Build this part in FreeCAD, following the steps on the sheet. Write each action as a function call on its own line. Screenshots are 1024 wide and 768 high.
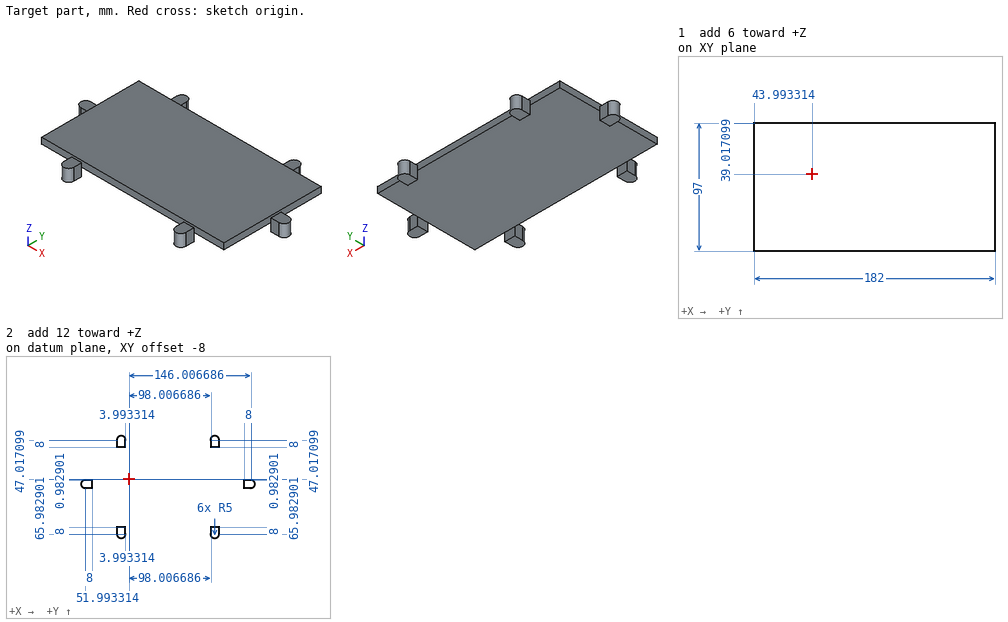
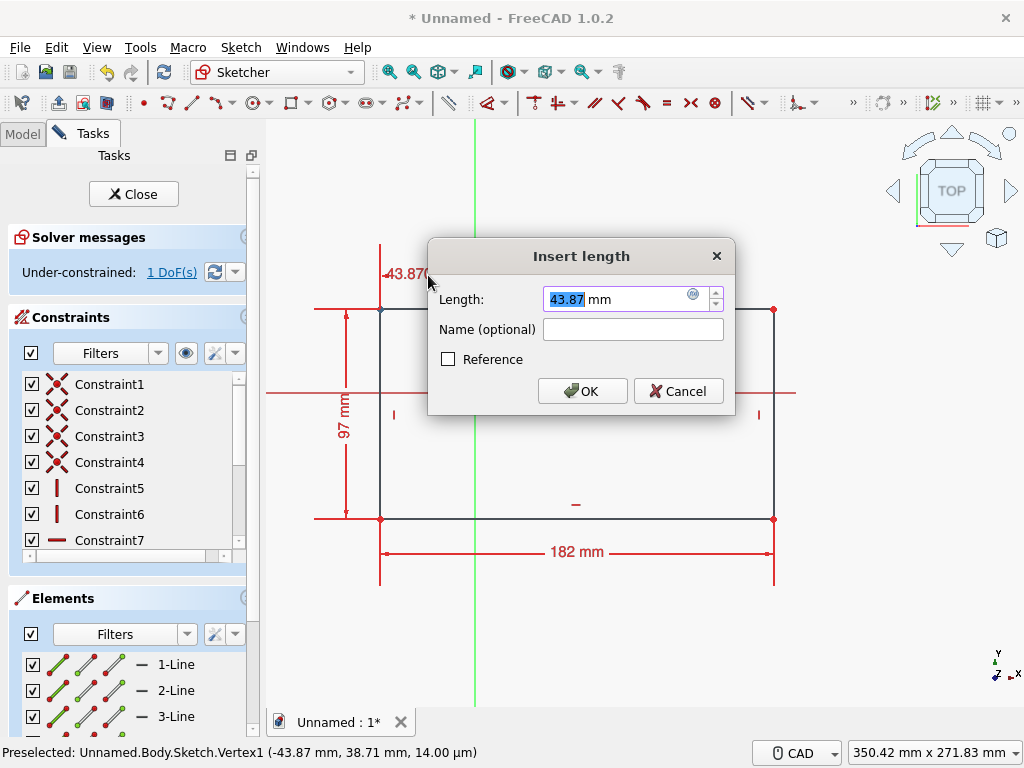
text(43.993314)
key(Return)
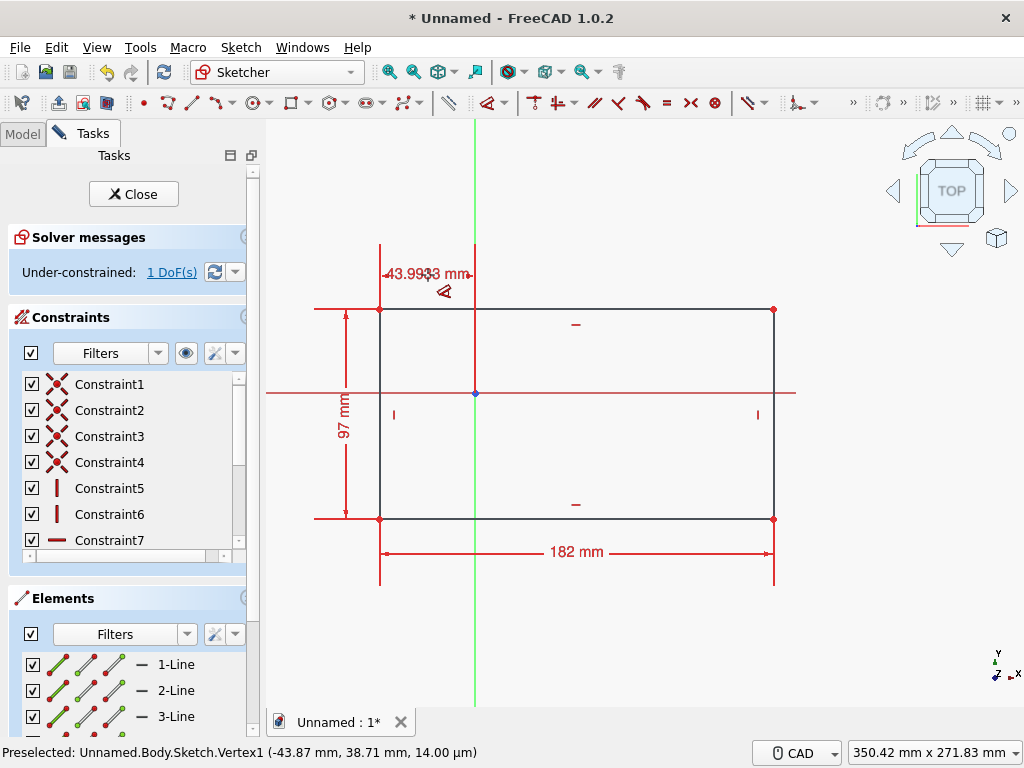
click(380, 309)
click(346, 351)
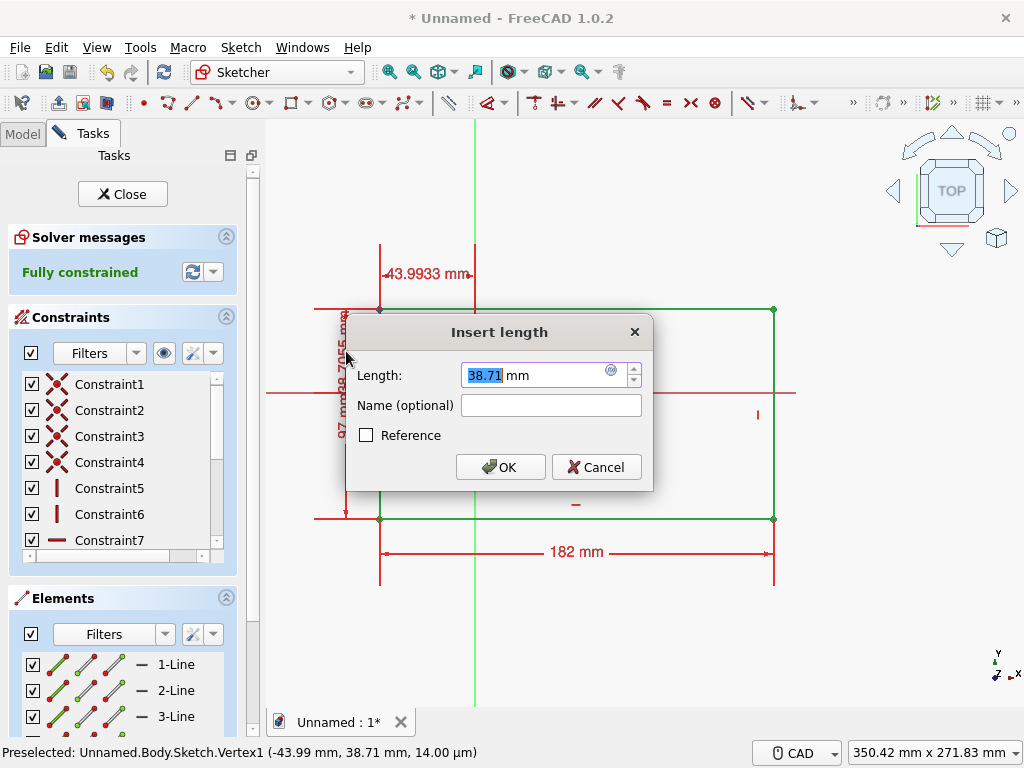
text(39.017099)
key(Return)
key(Escape)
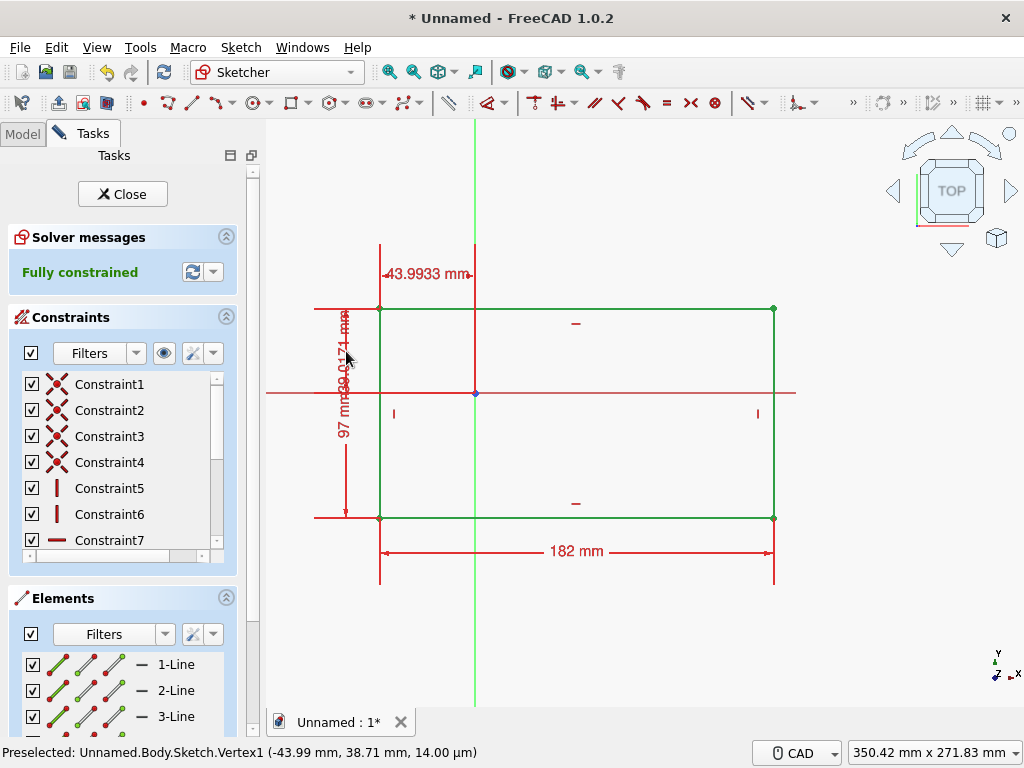
click(123, 194)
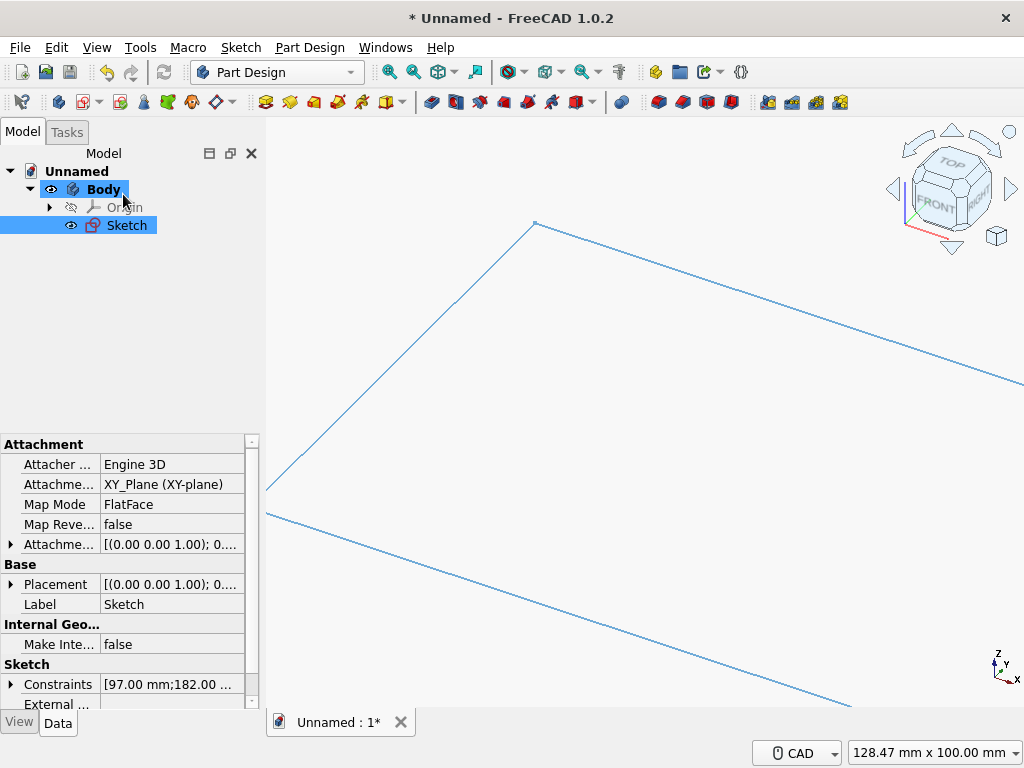
click(266, 102)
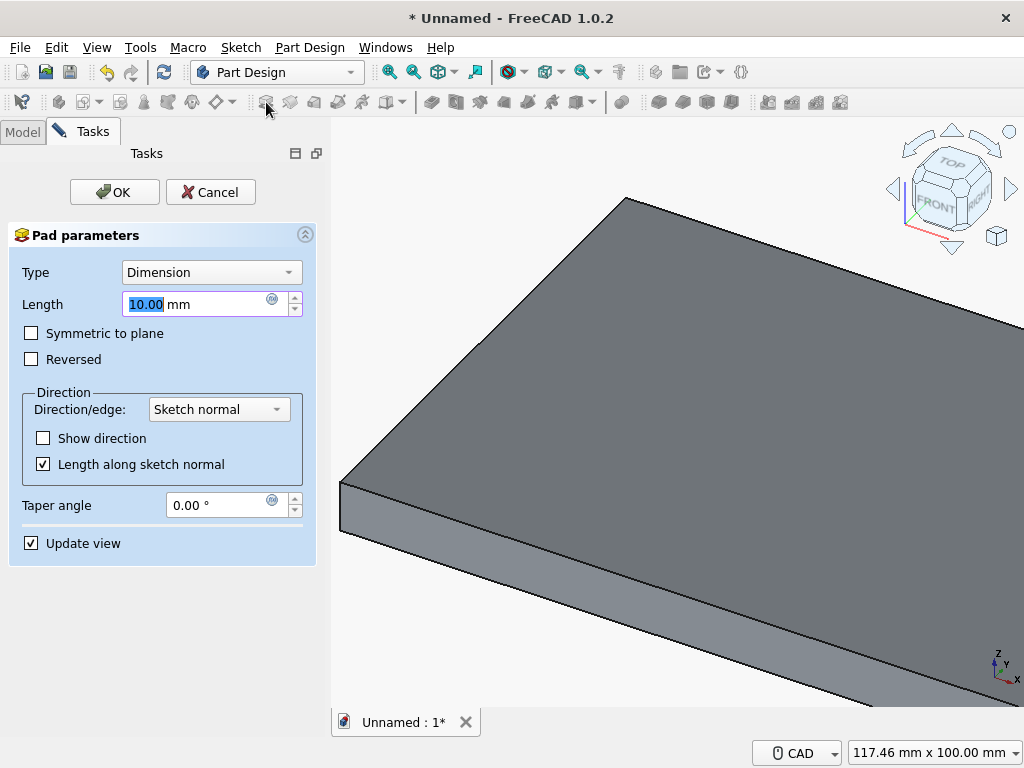
text(6)
key(Tab)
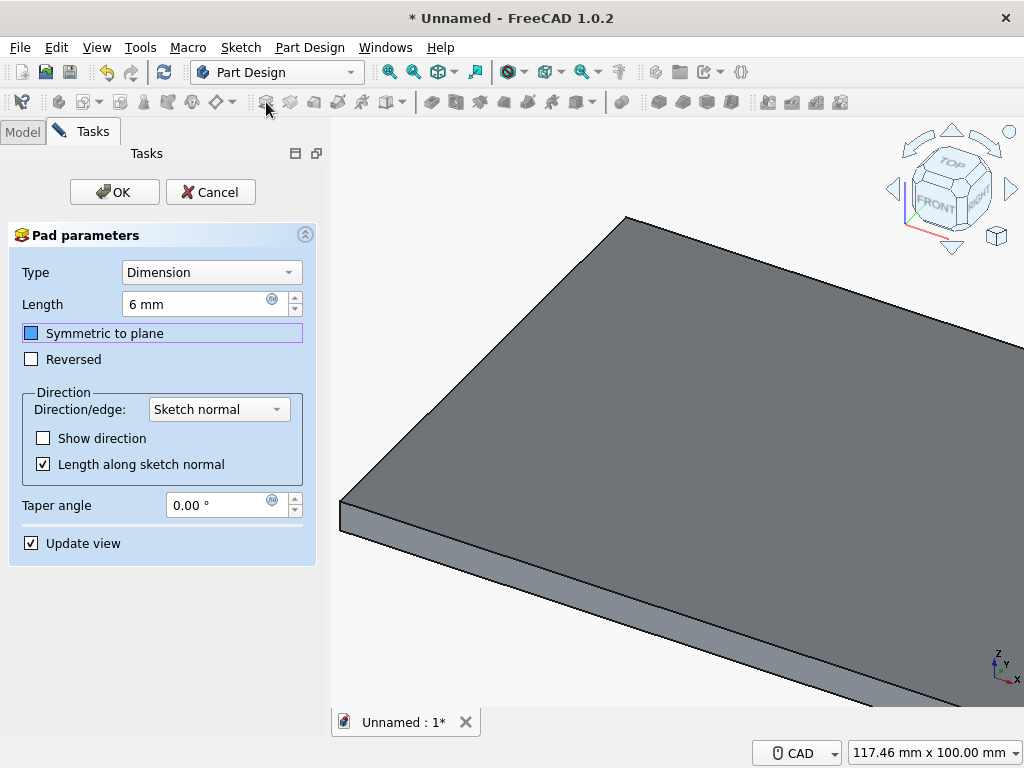
click(115, 192)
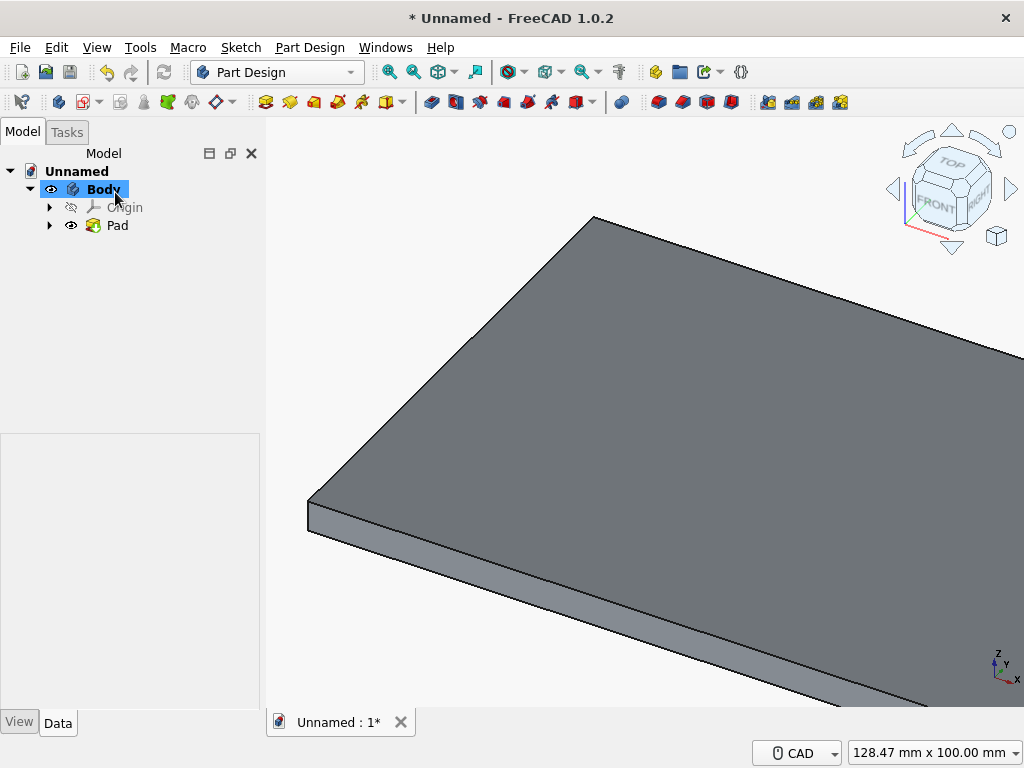
click(390, 72)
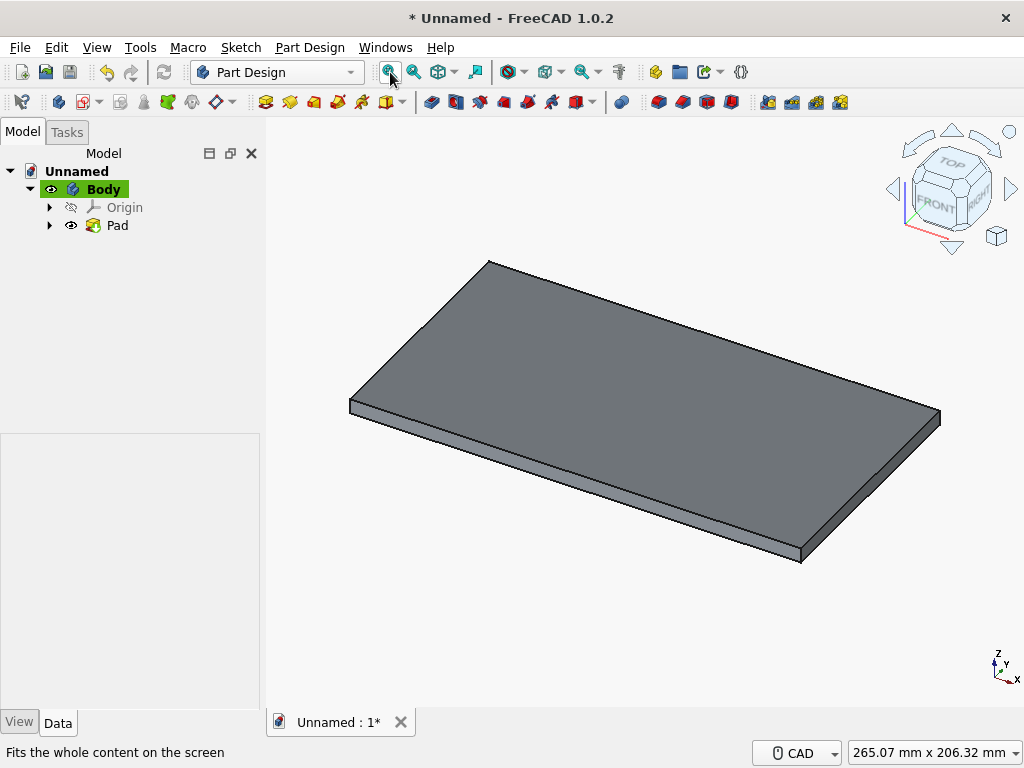
click(50, 207)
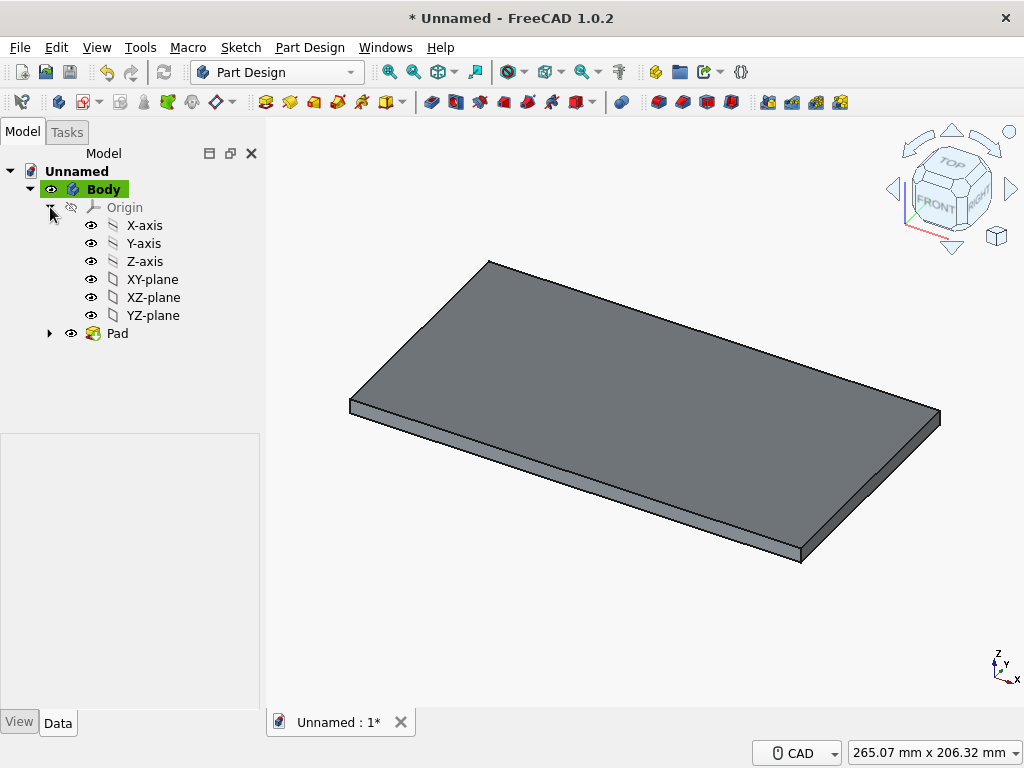
click(136, 279)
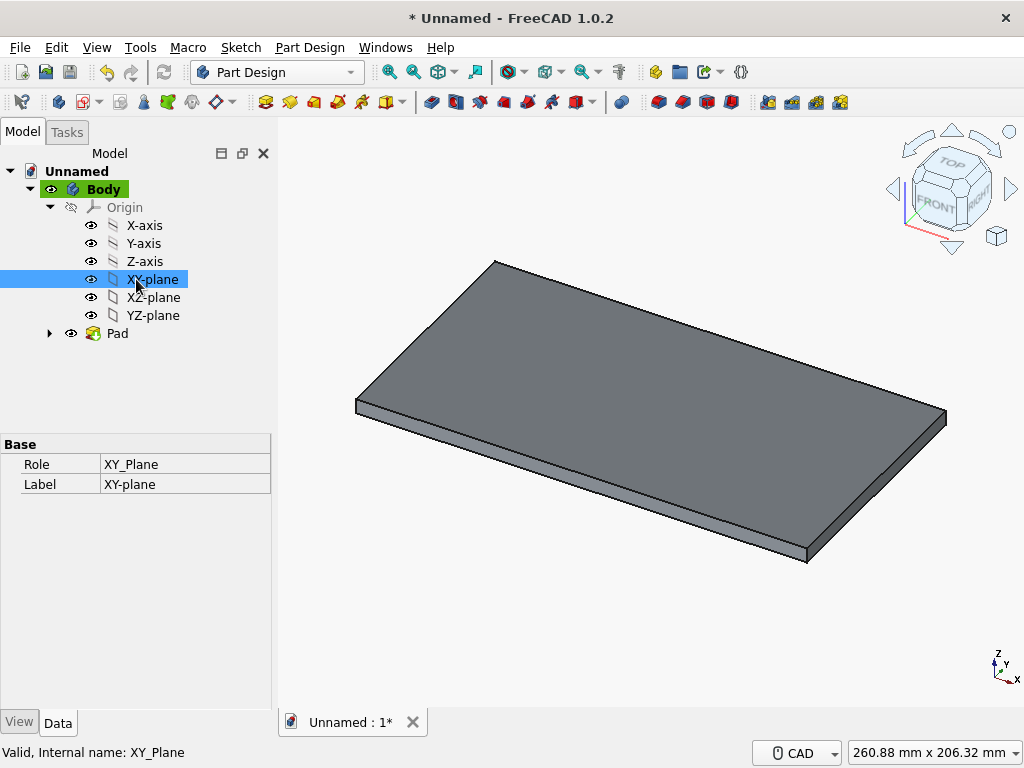
click(216, 102)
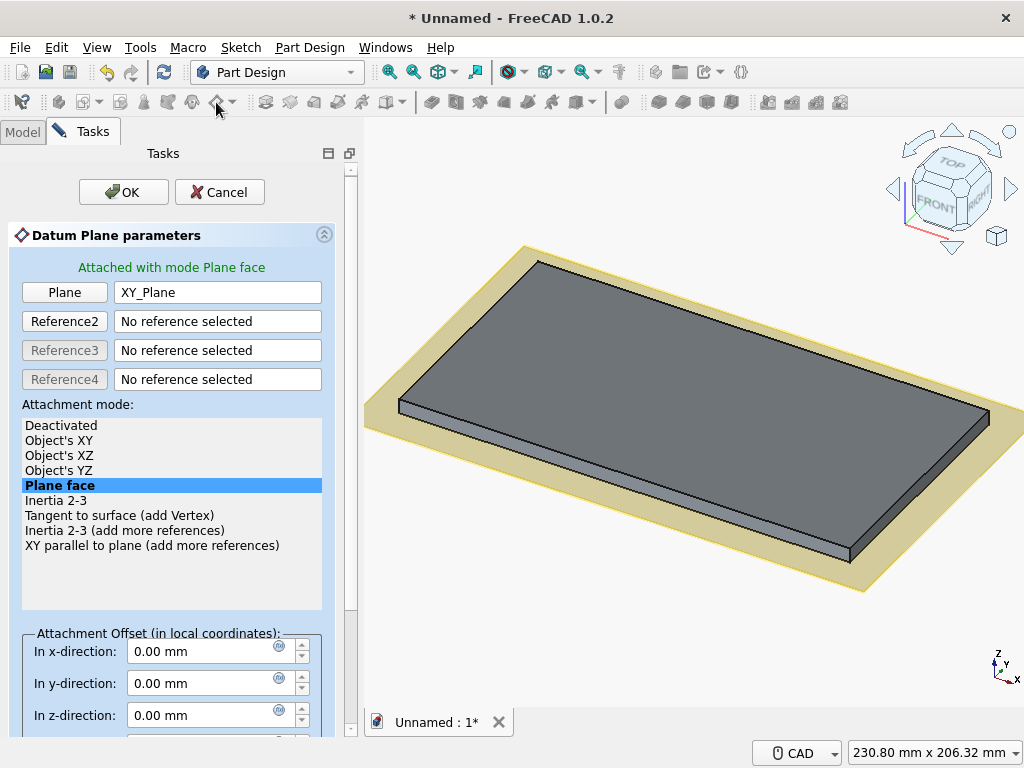
triple_click(210, 715)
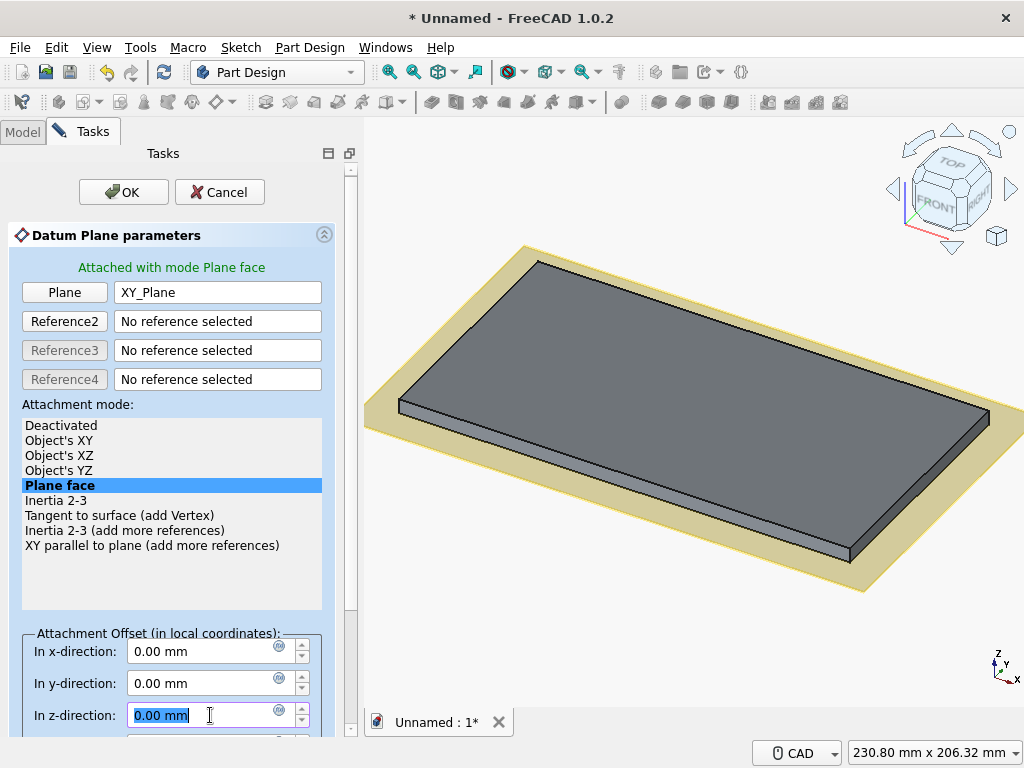
text(-8)
key(Tab)